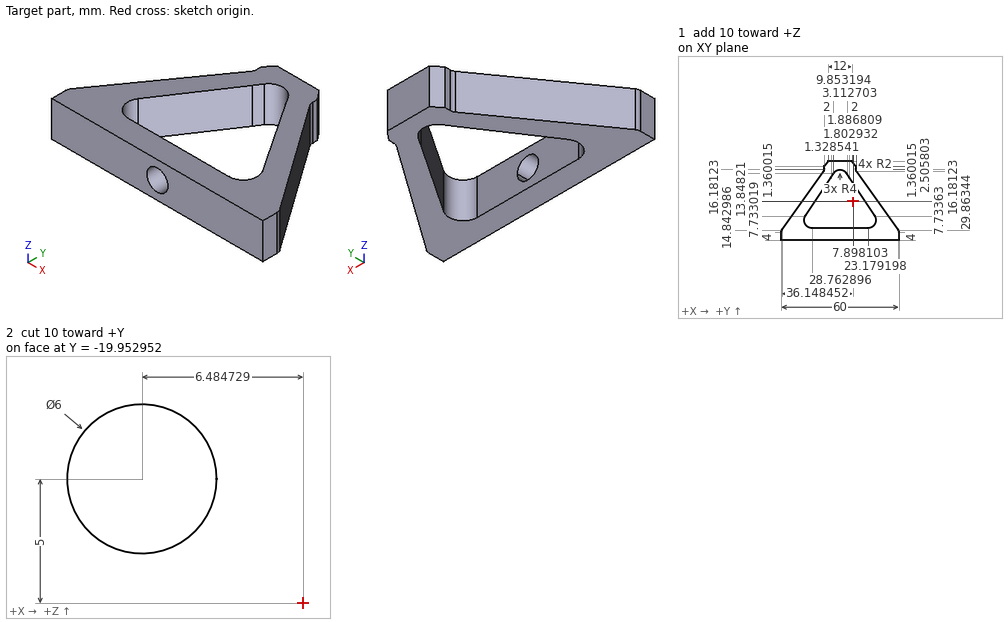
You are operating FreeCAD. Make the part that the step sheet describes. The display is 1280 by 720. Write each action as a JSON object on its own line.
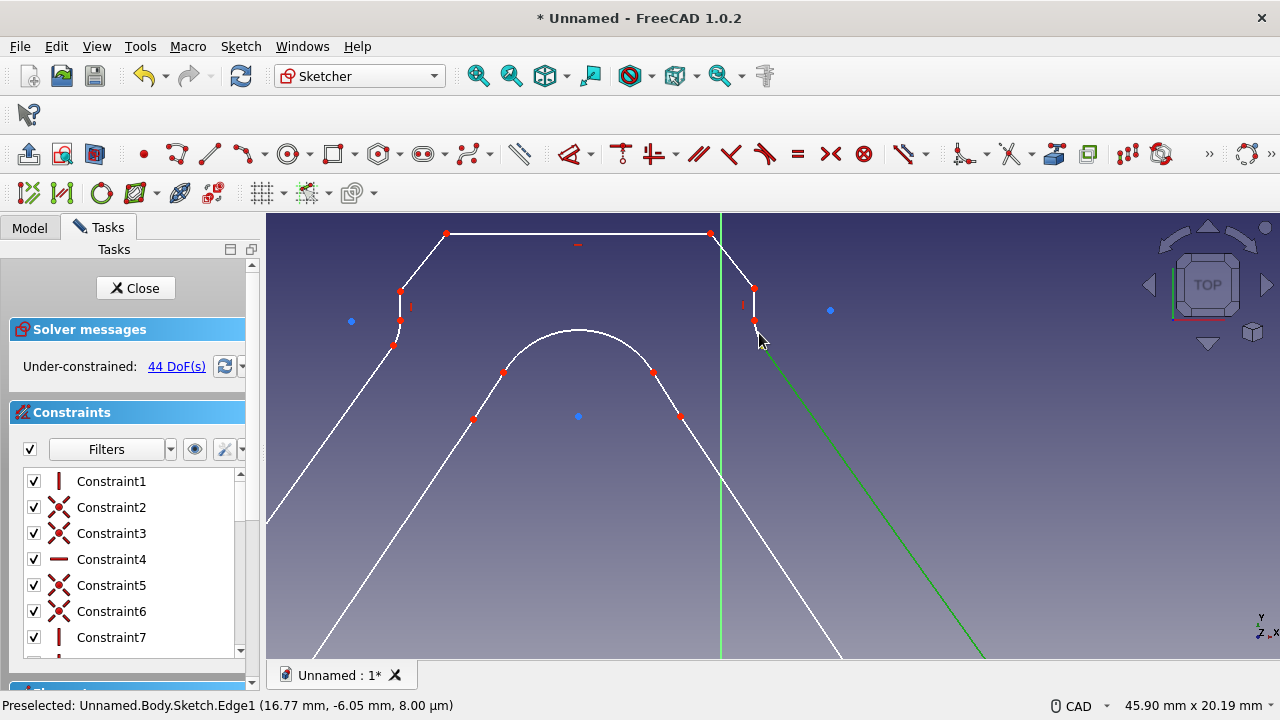
{"action": "left_click", "coordinate": [757, 333]}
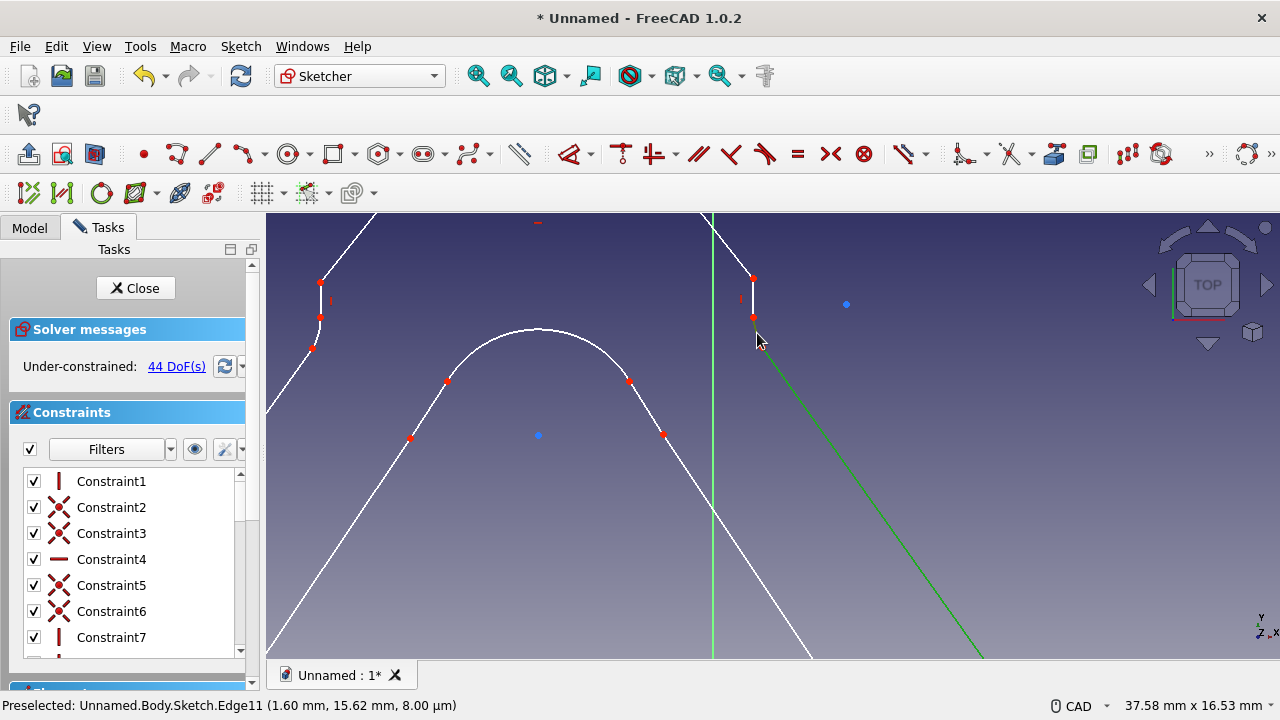
{"action": "left_click", "coordinate": [765, 154]}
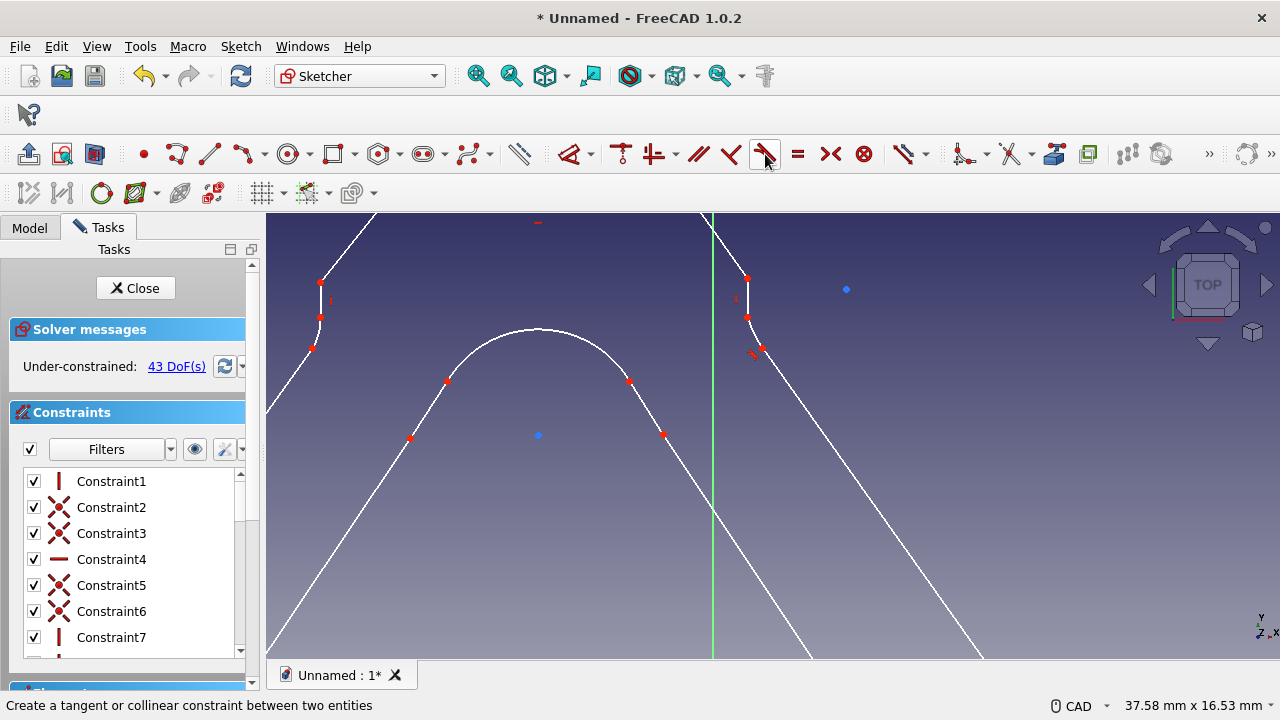
{"action": "left_click", "coordinate": [748, 306]}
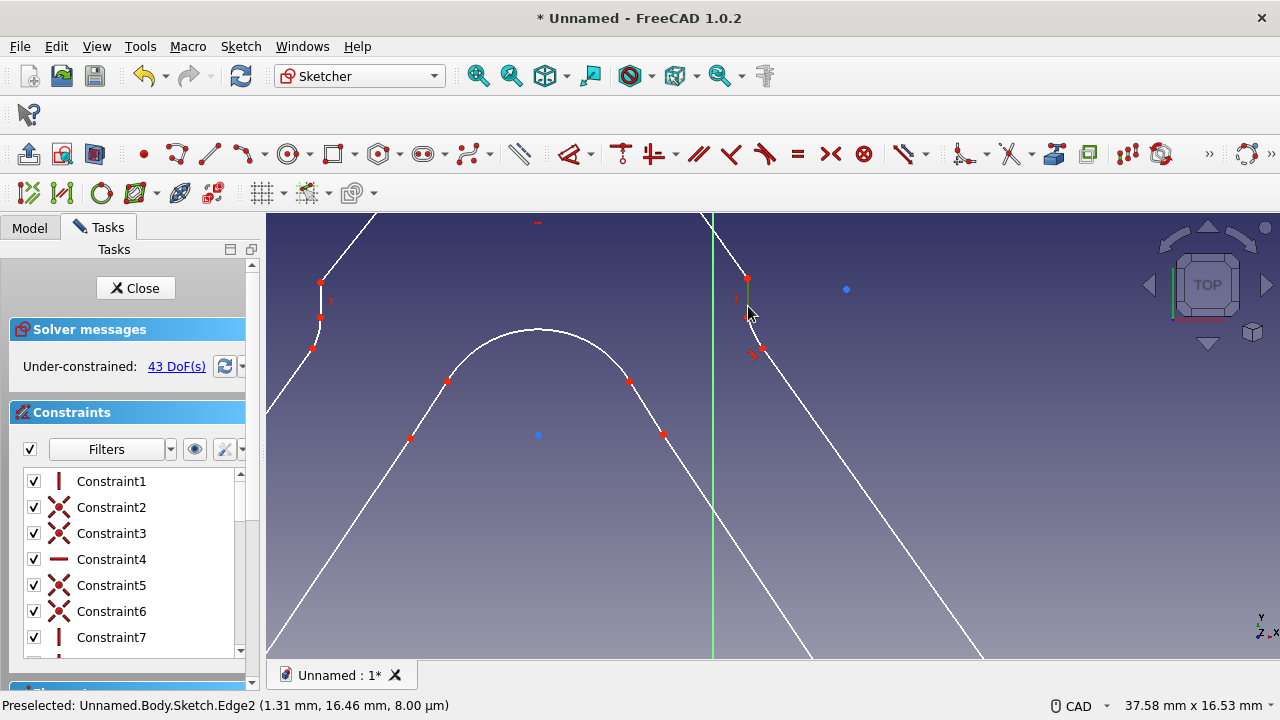
{"action": "scroll", "coordinate": [751, 327], "scroll_direction": "up", "scroll_amount": 2}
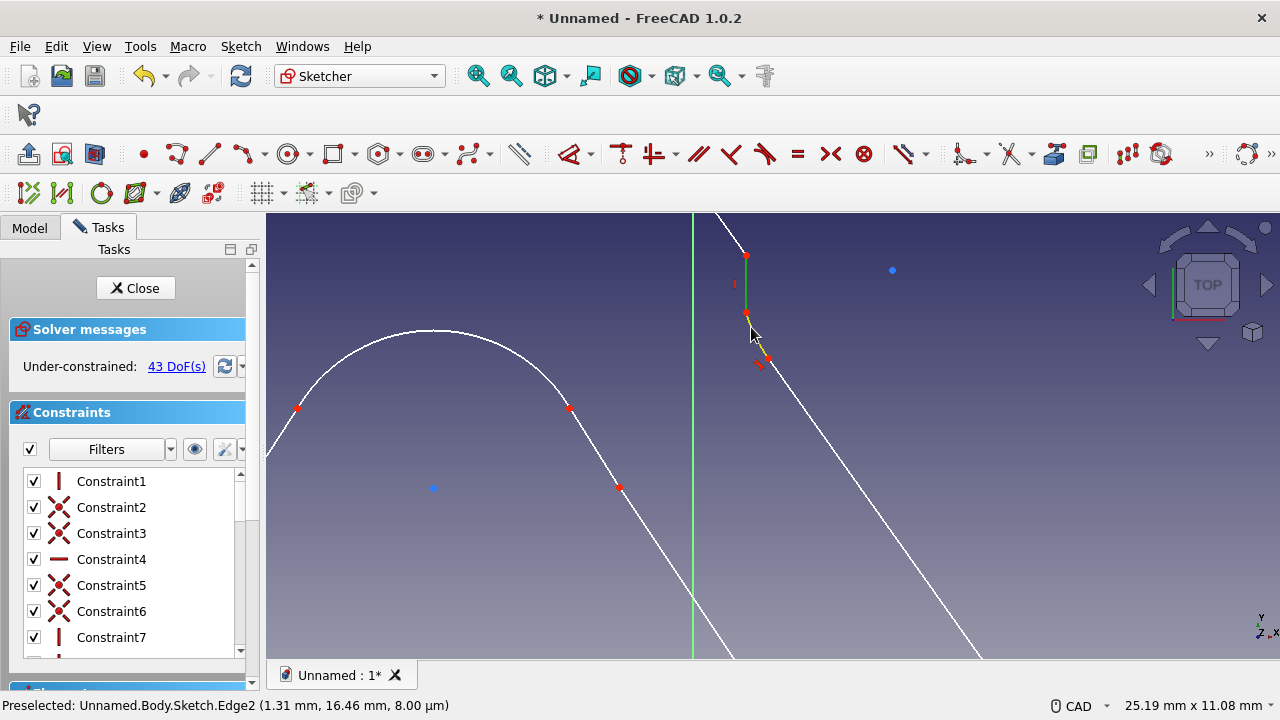
{"action": "left_click", "coordinate": [751, 327]}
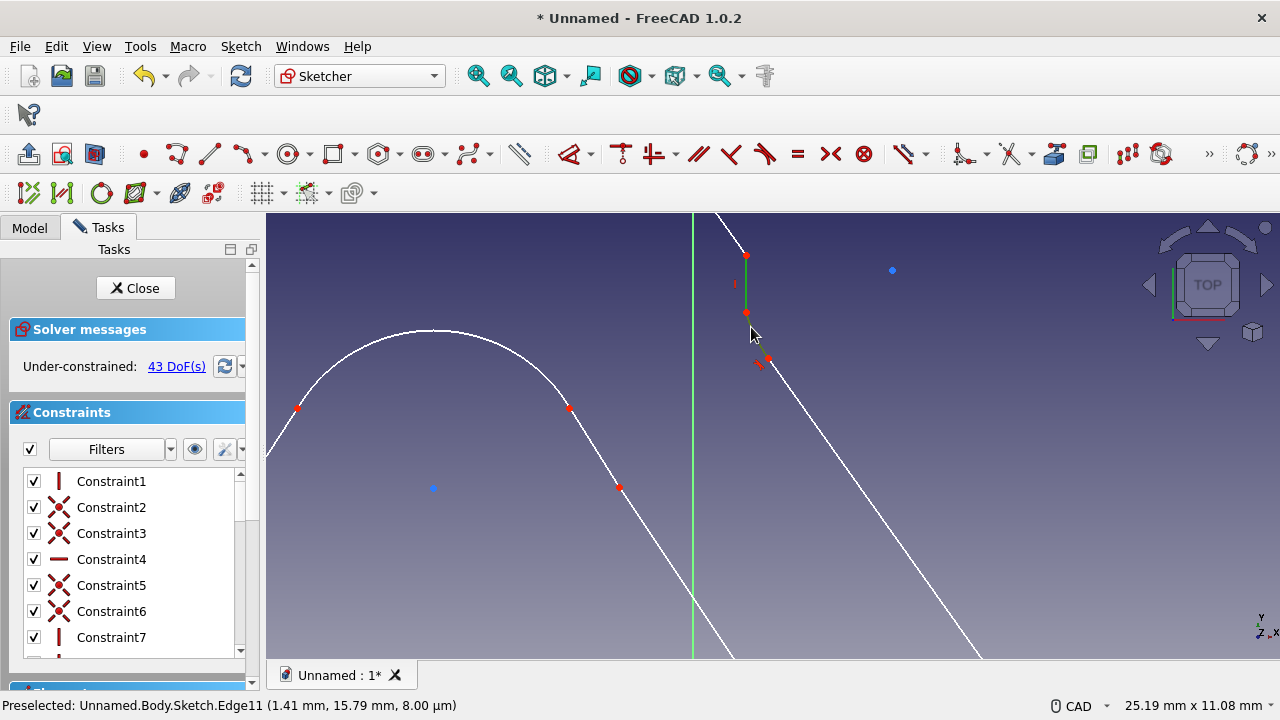
{"action": "left_click", "coordinate": [765, 154]}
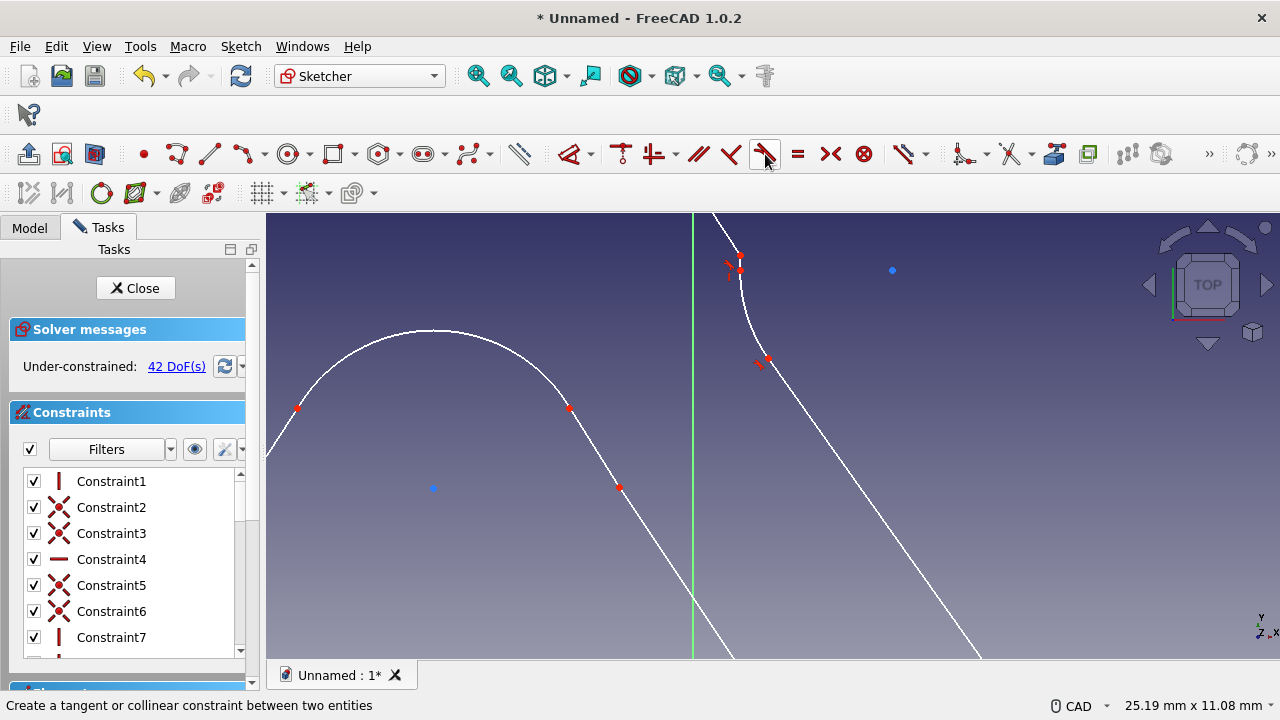
{"action": "scroll", "coordinate": [758, 333], "scroll_direction": "down", "scroll_amount": 9}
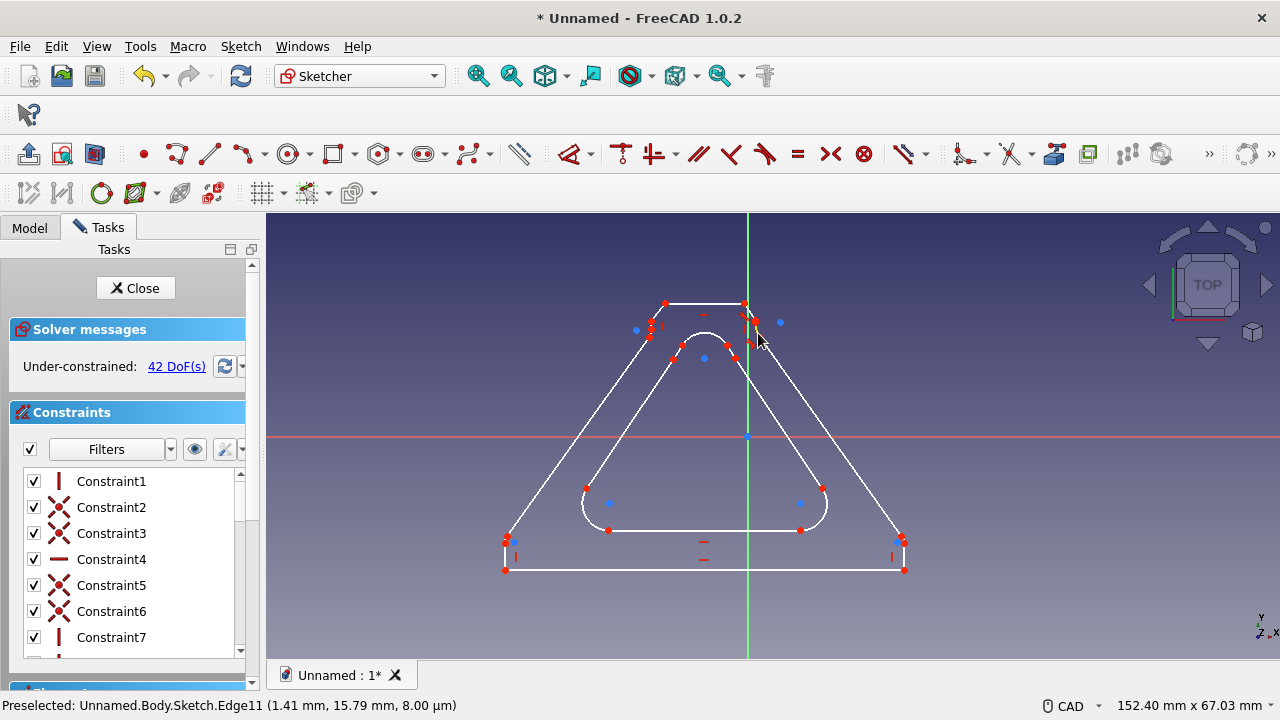
{"action": "scroll", "coordinate": [651, 324], "scroll_direction": "up", "scroll_amount": 9}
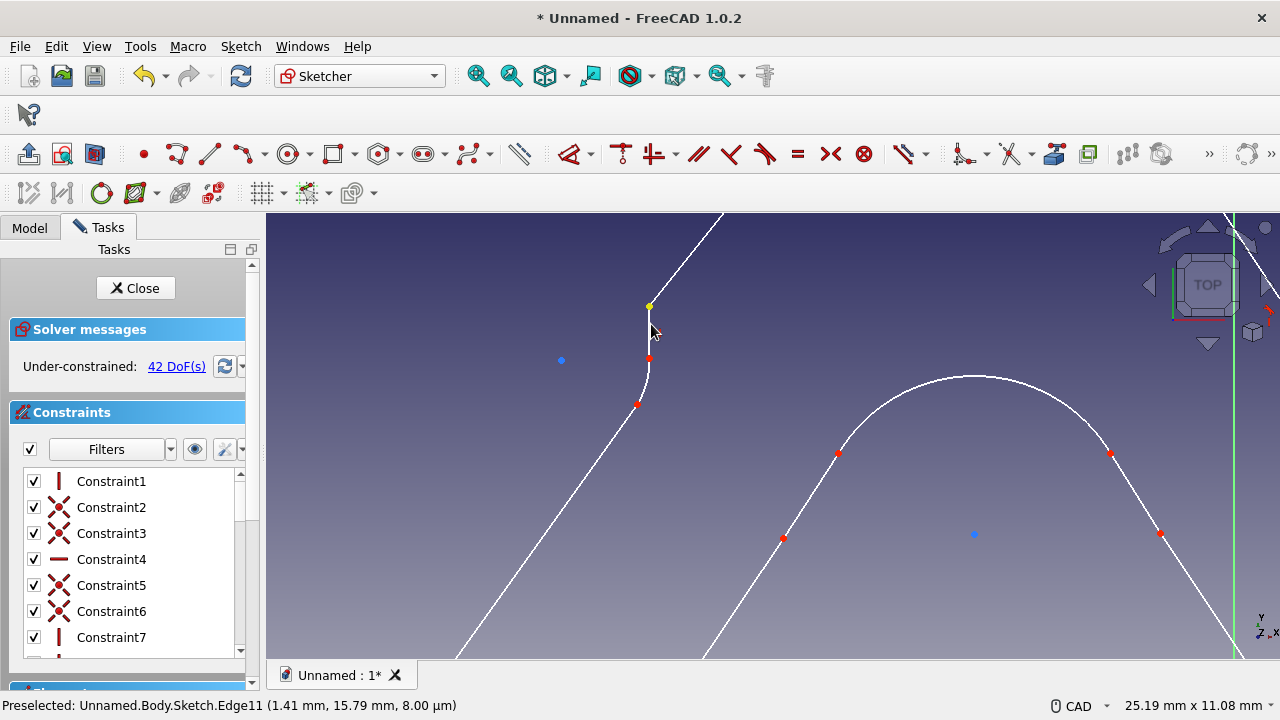
{"action": "left_click", "coordinate": [649, 322]}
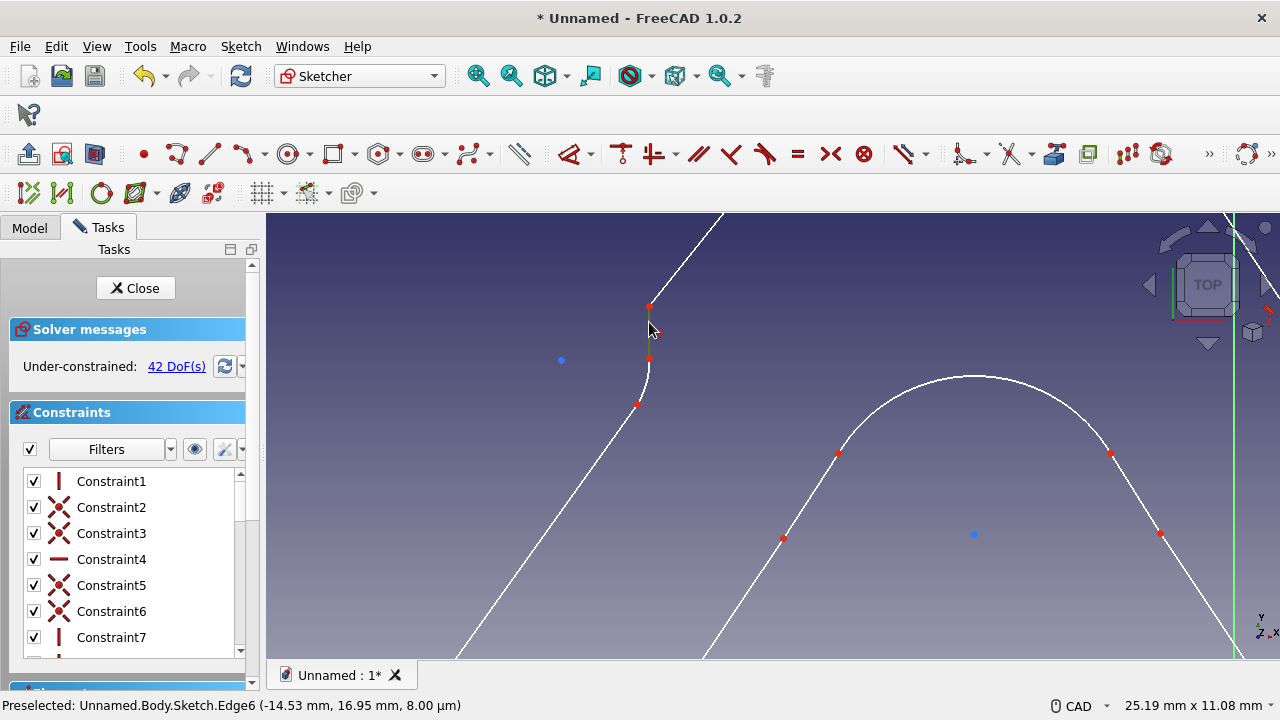
{"action": "left_click", "coordinate": [644, 392]}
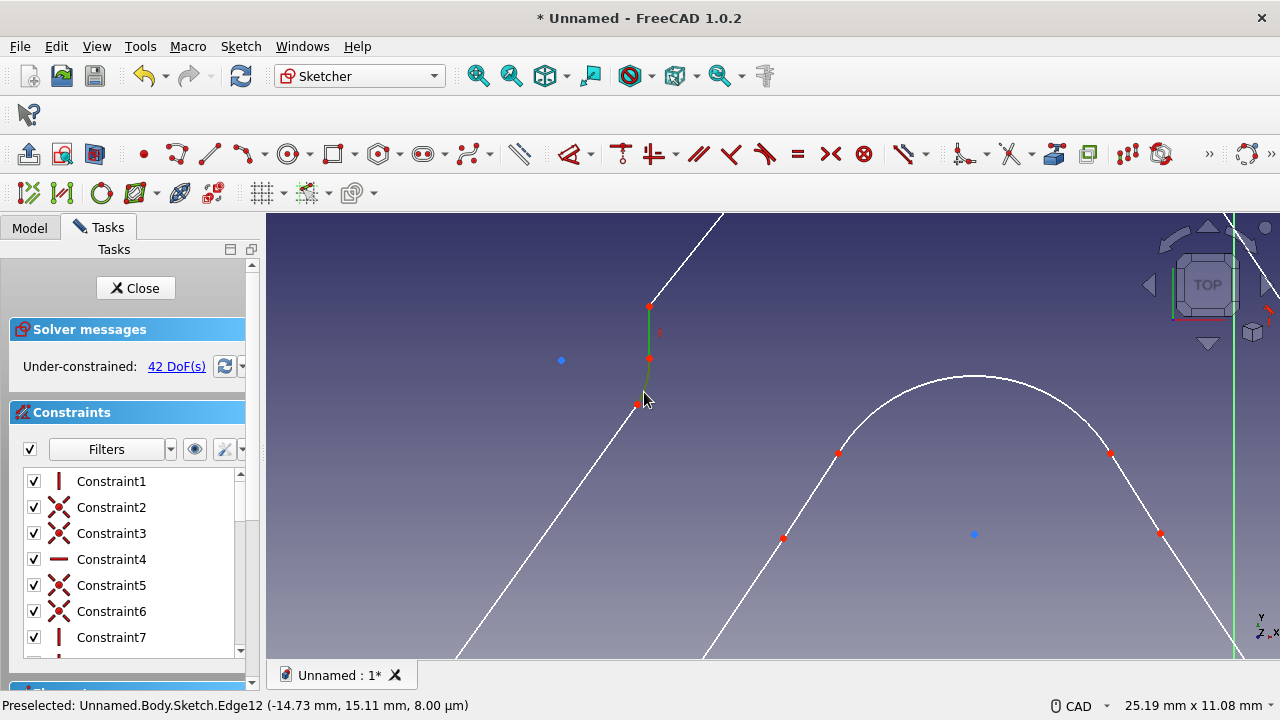
{"action": "left_click", "coordinate": [765, 154]}